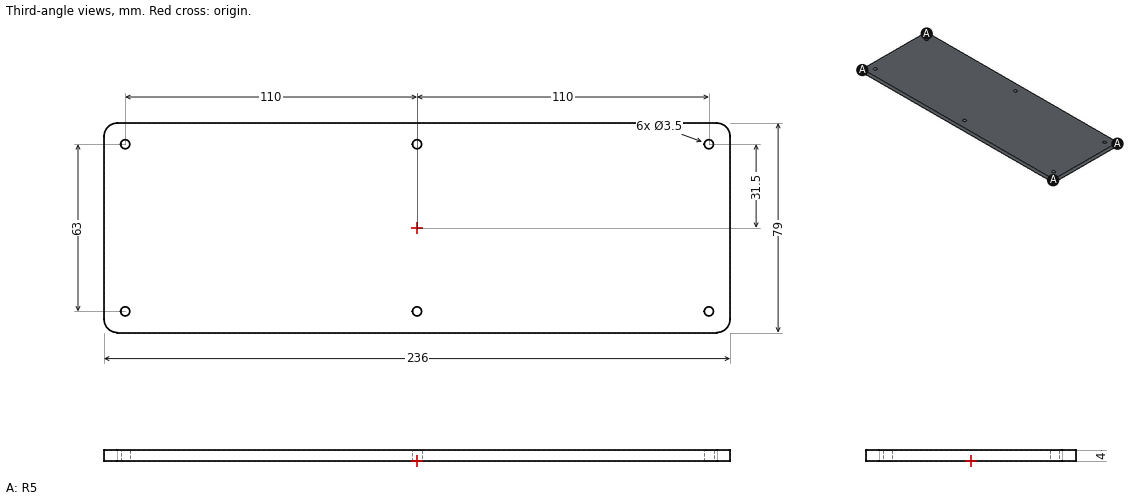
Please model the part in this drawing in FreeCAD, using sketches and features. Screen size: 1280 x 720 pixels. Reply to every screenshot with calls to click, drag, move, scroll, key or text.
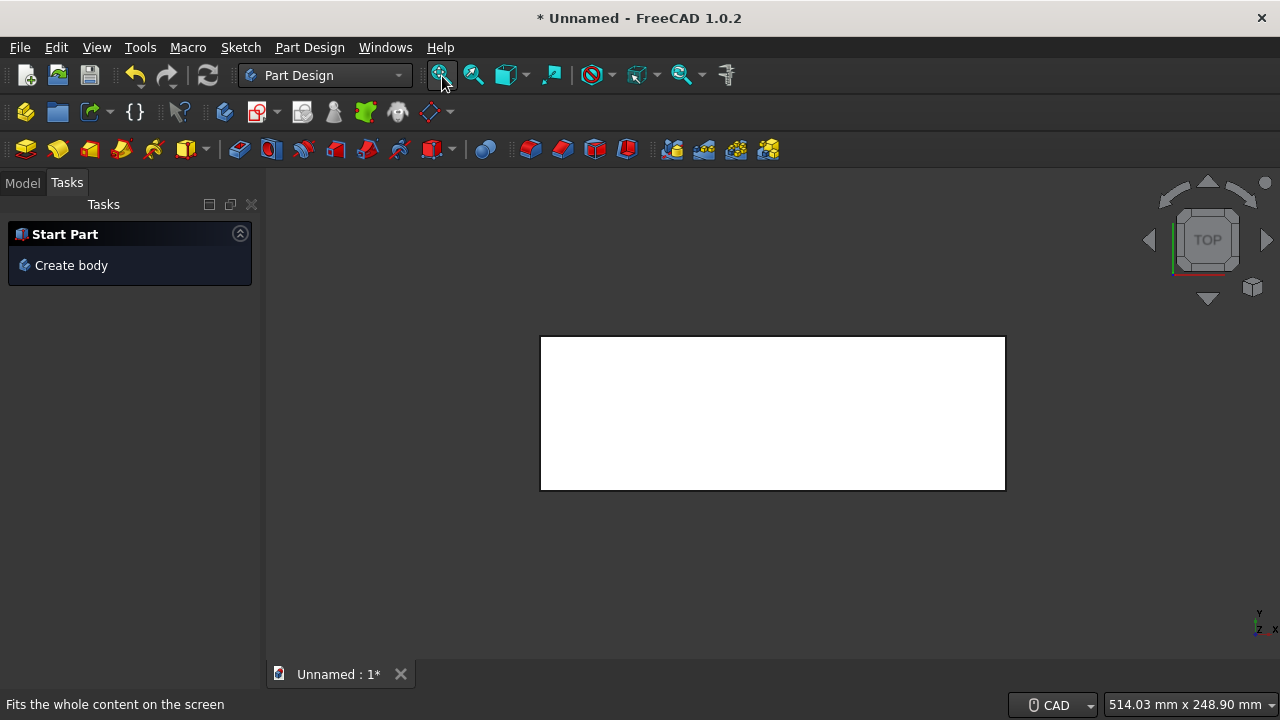
scroll(540, 412, up, 9)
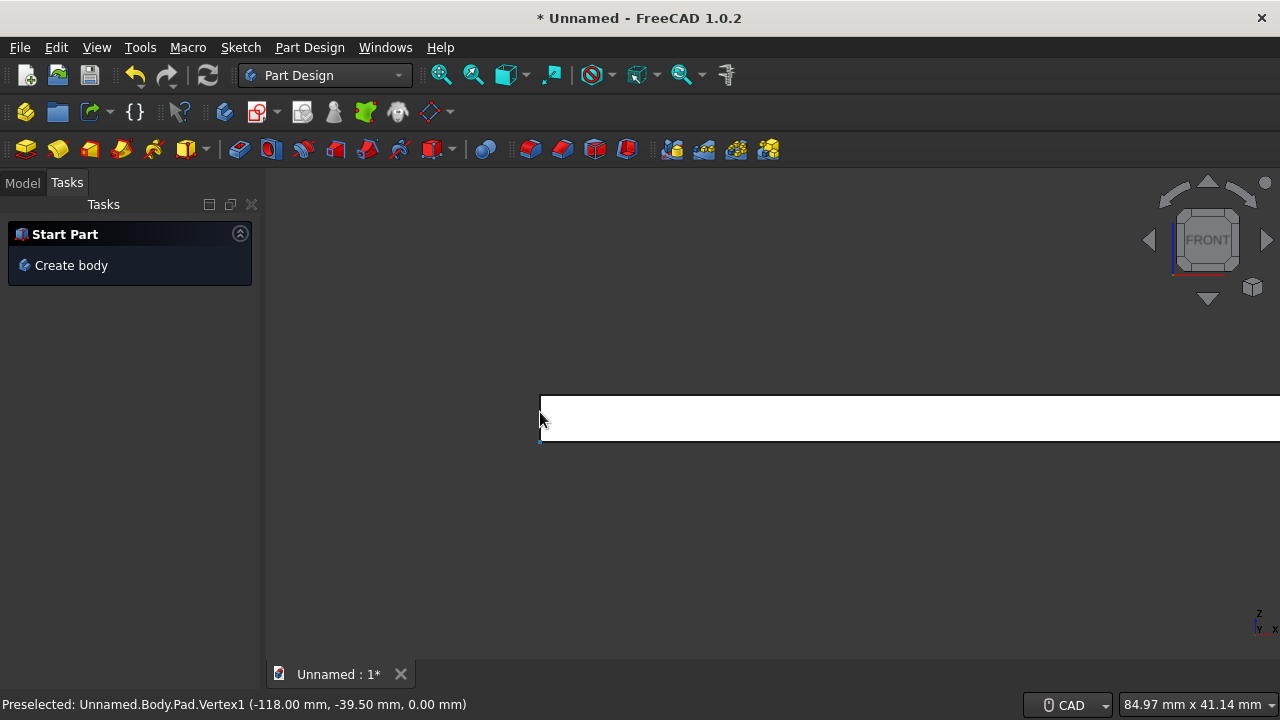
click(540, 418)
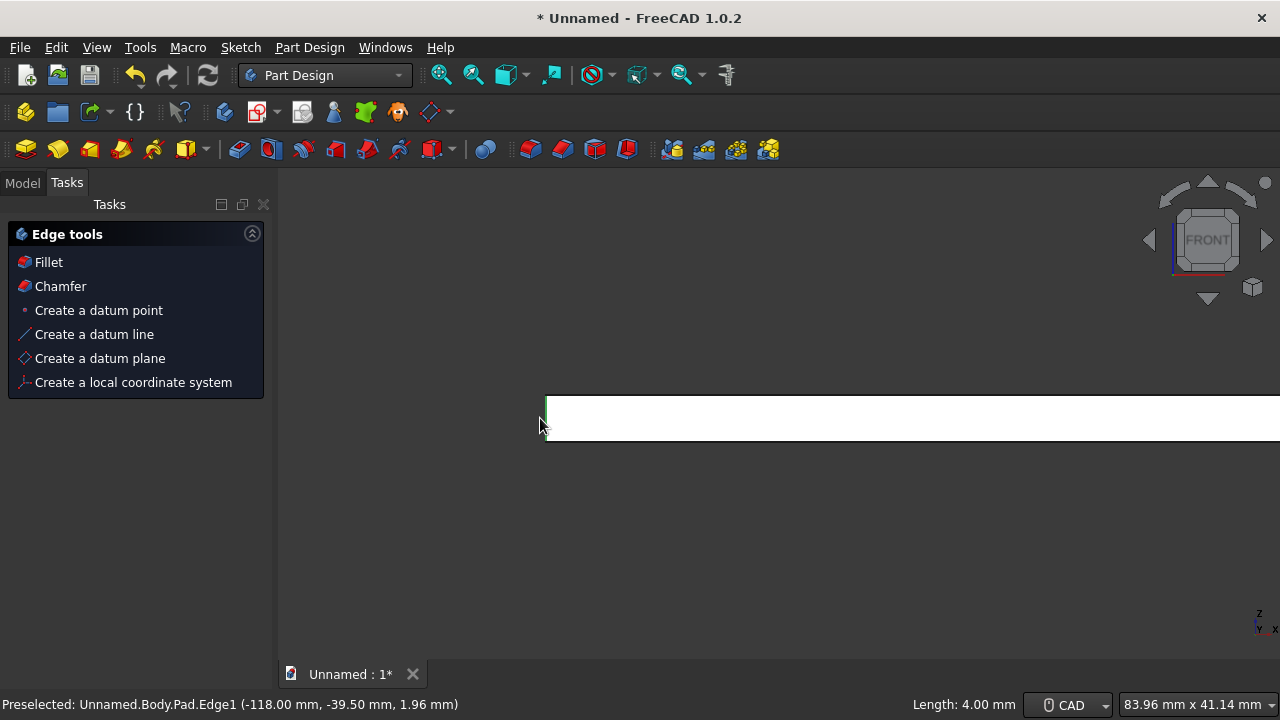
click(442, 76)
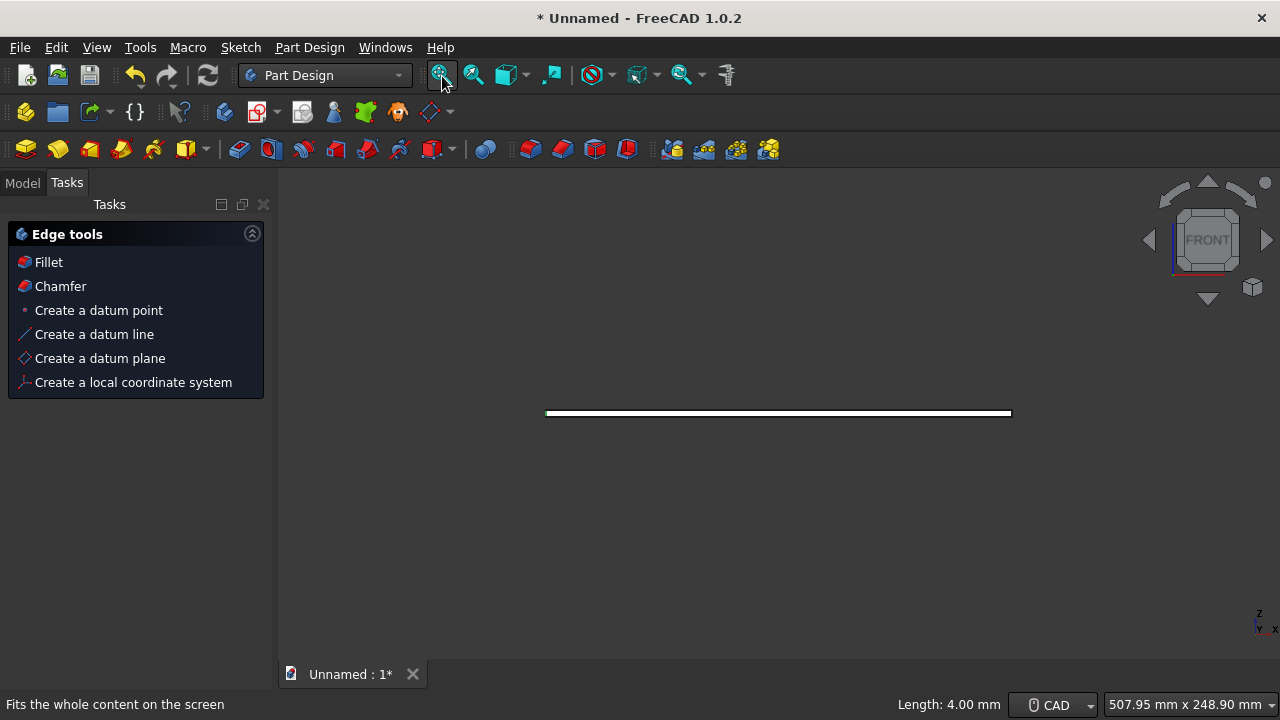
key(3)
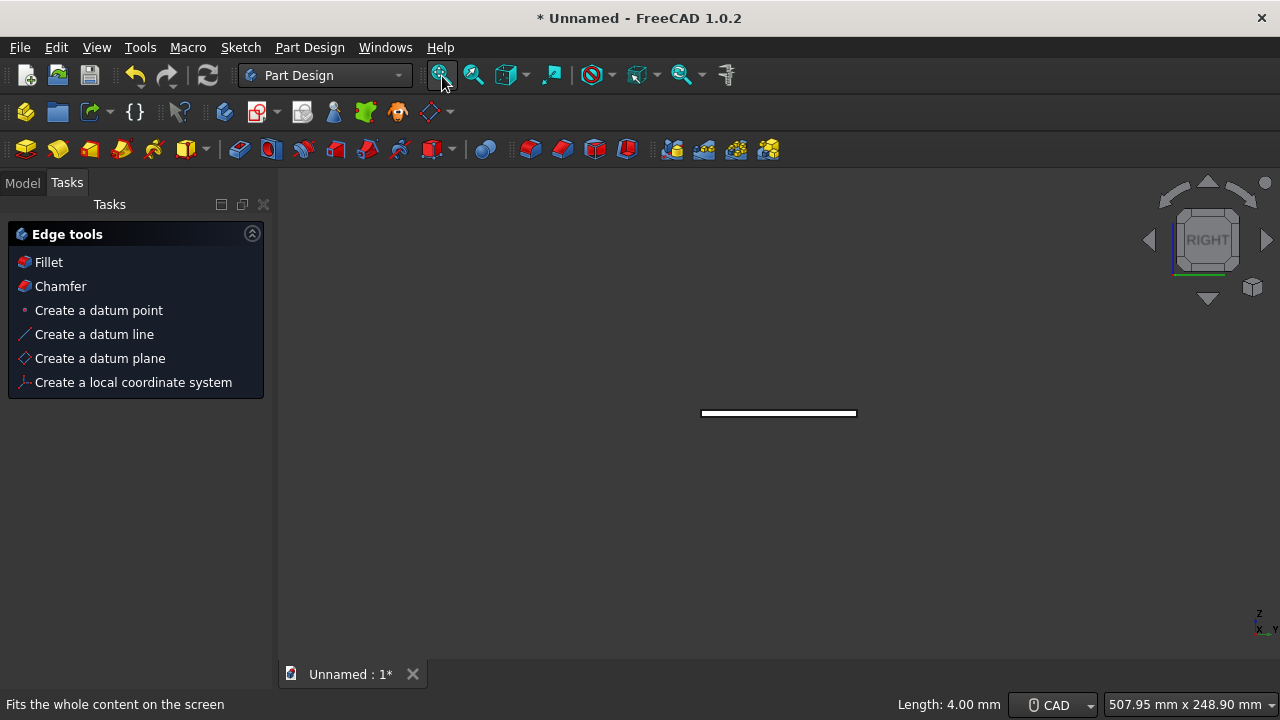
click(442, 76)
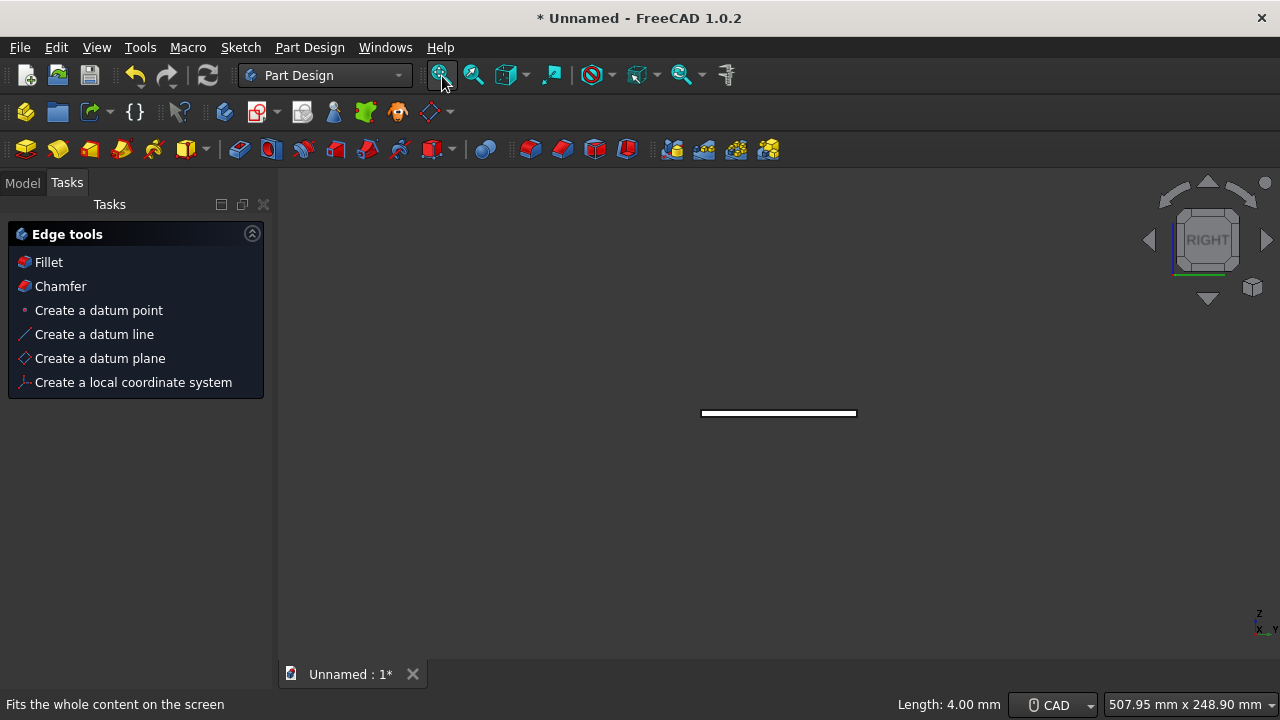
scroll(857, 412, up, 9)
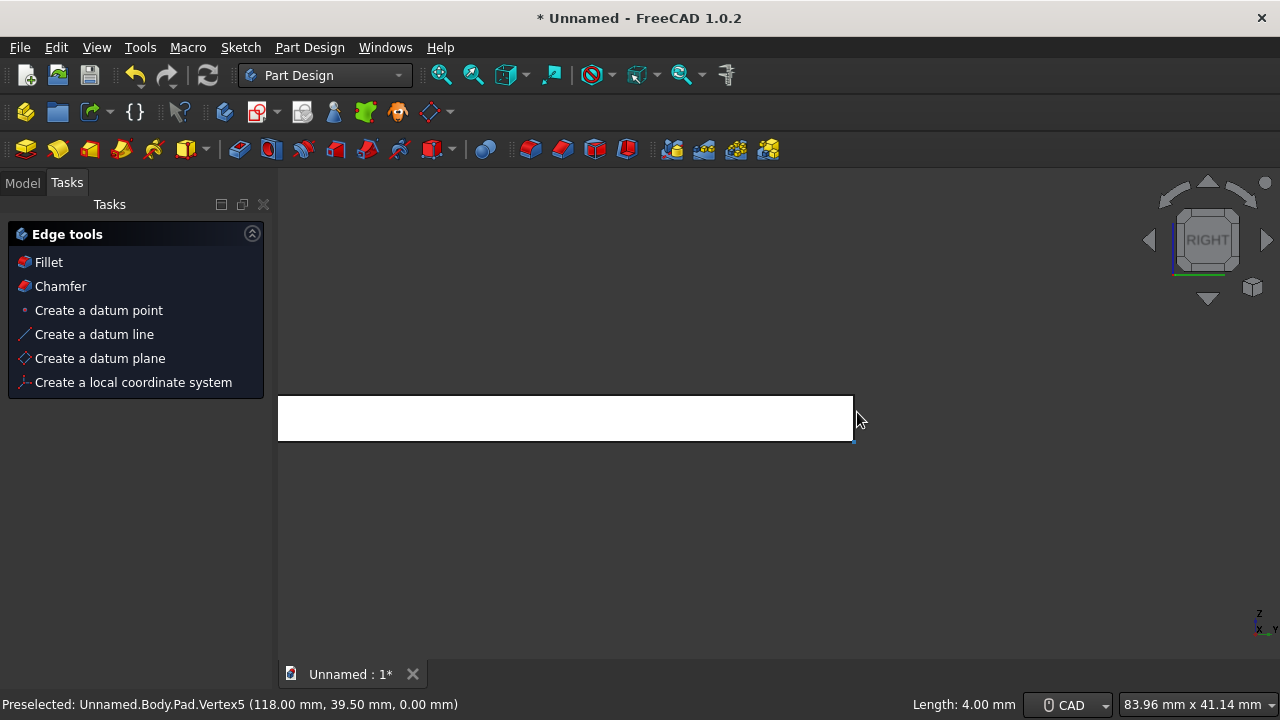
click(854, 418, ctrl)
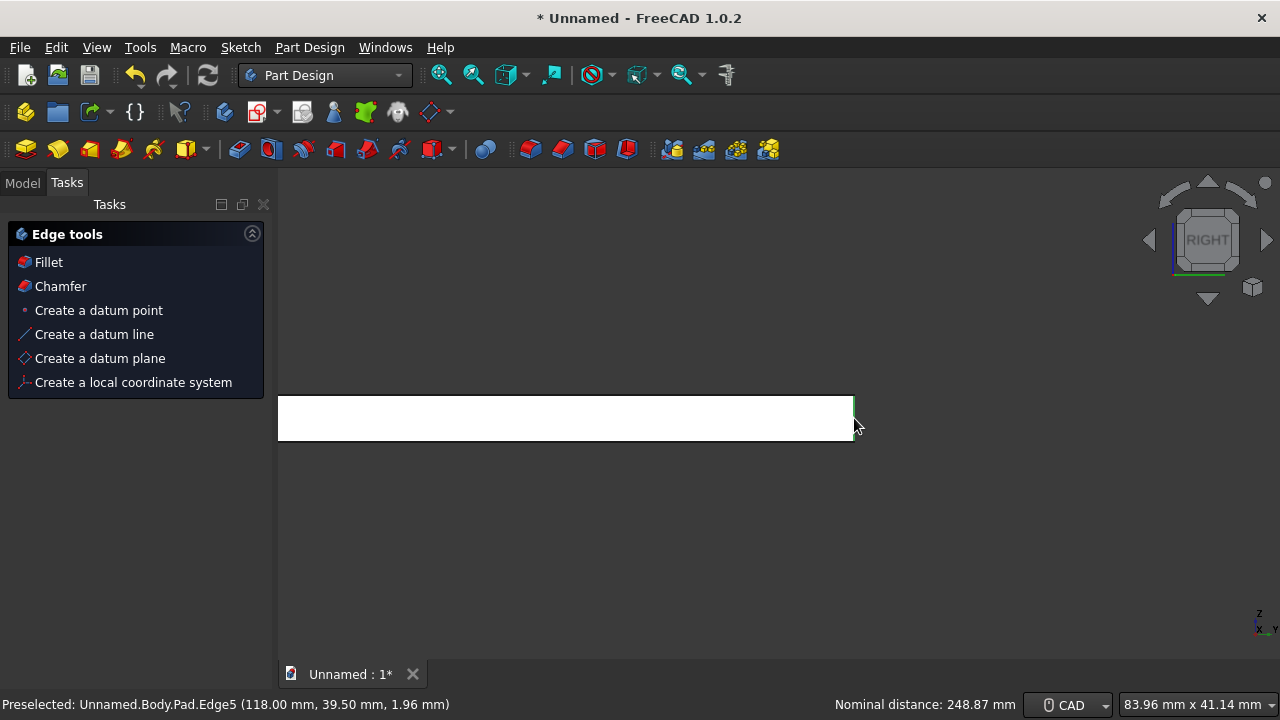
click(442, 76)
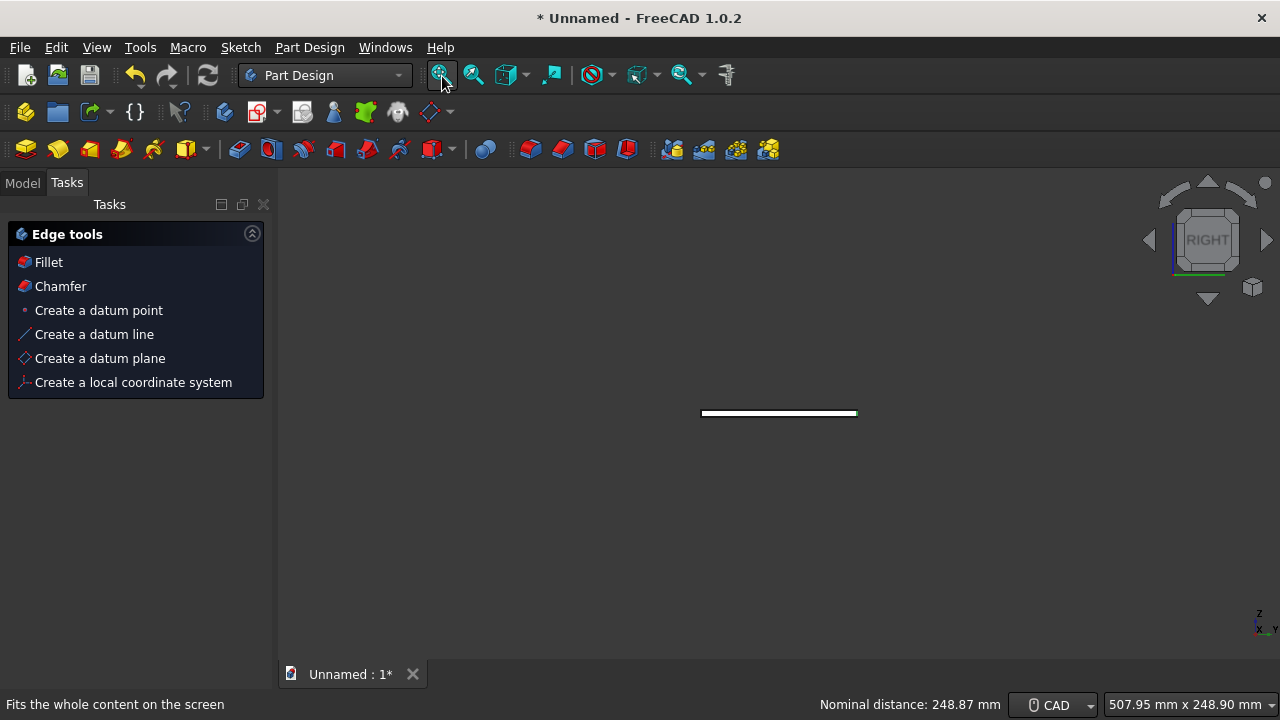
key(5)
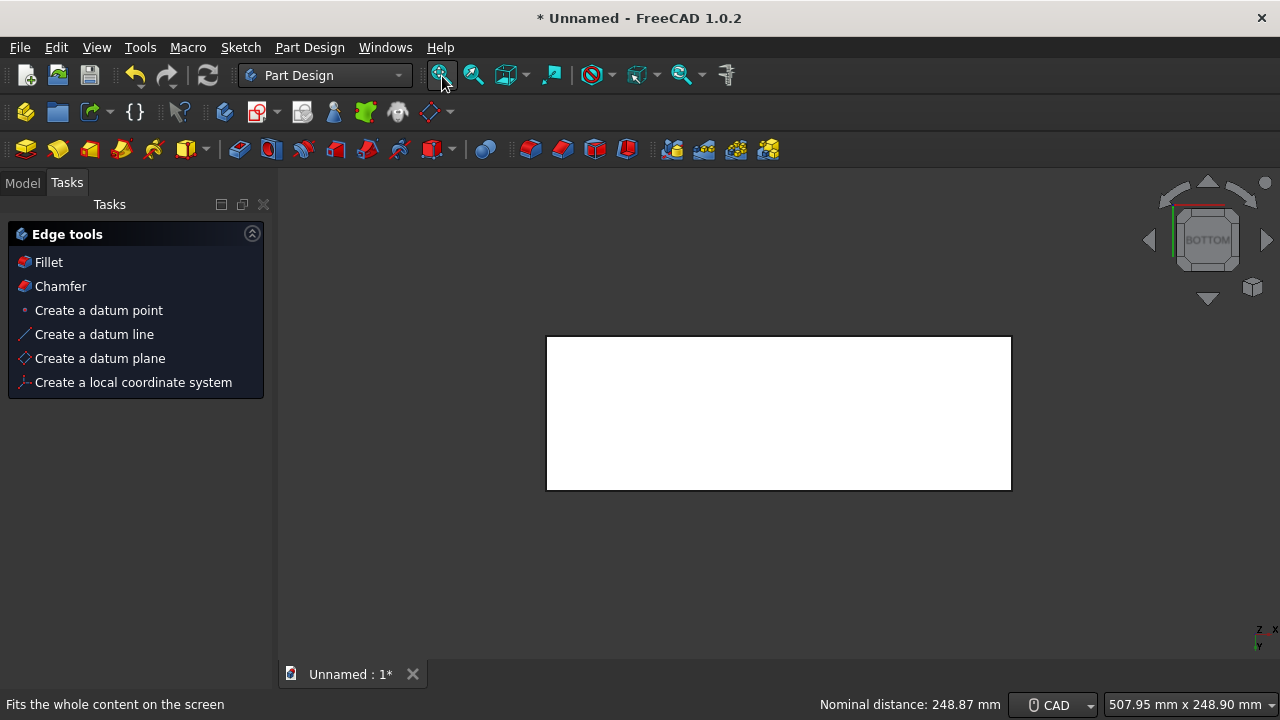
scroll(546, 490, up, 9)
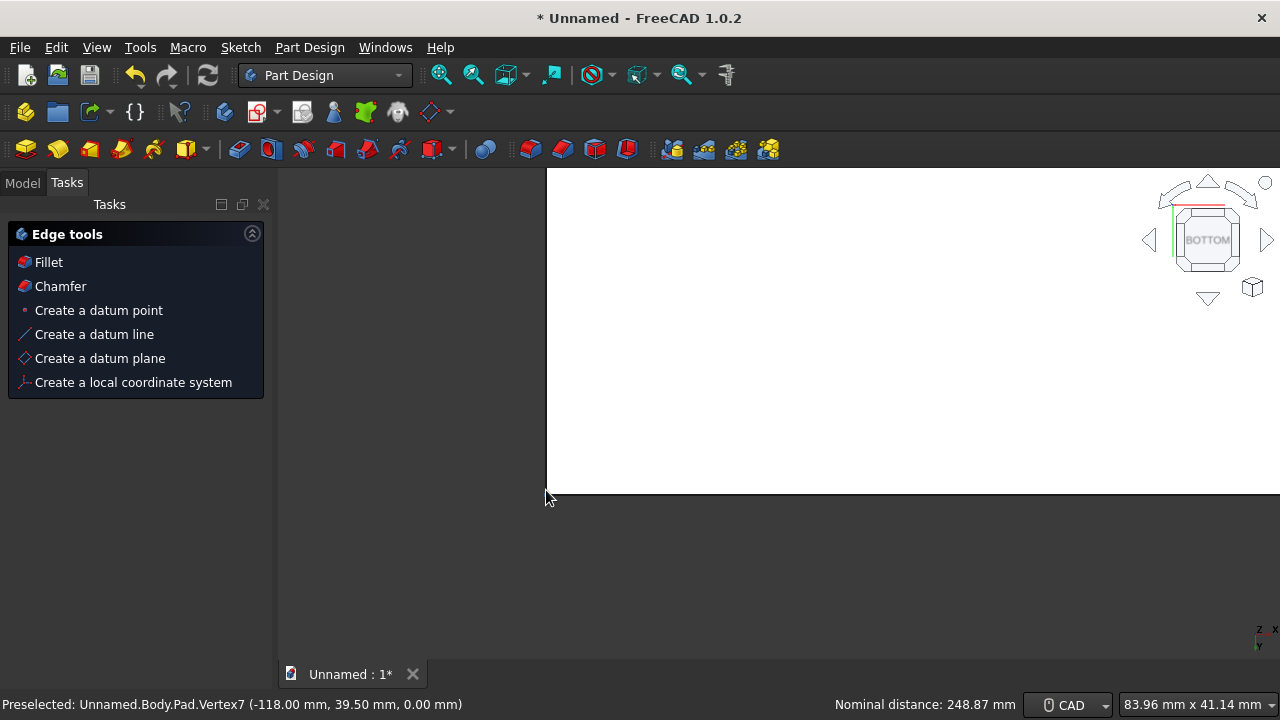
click(442, 76)